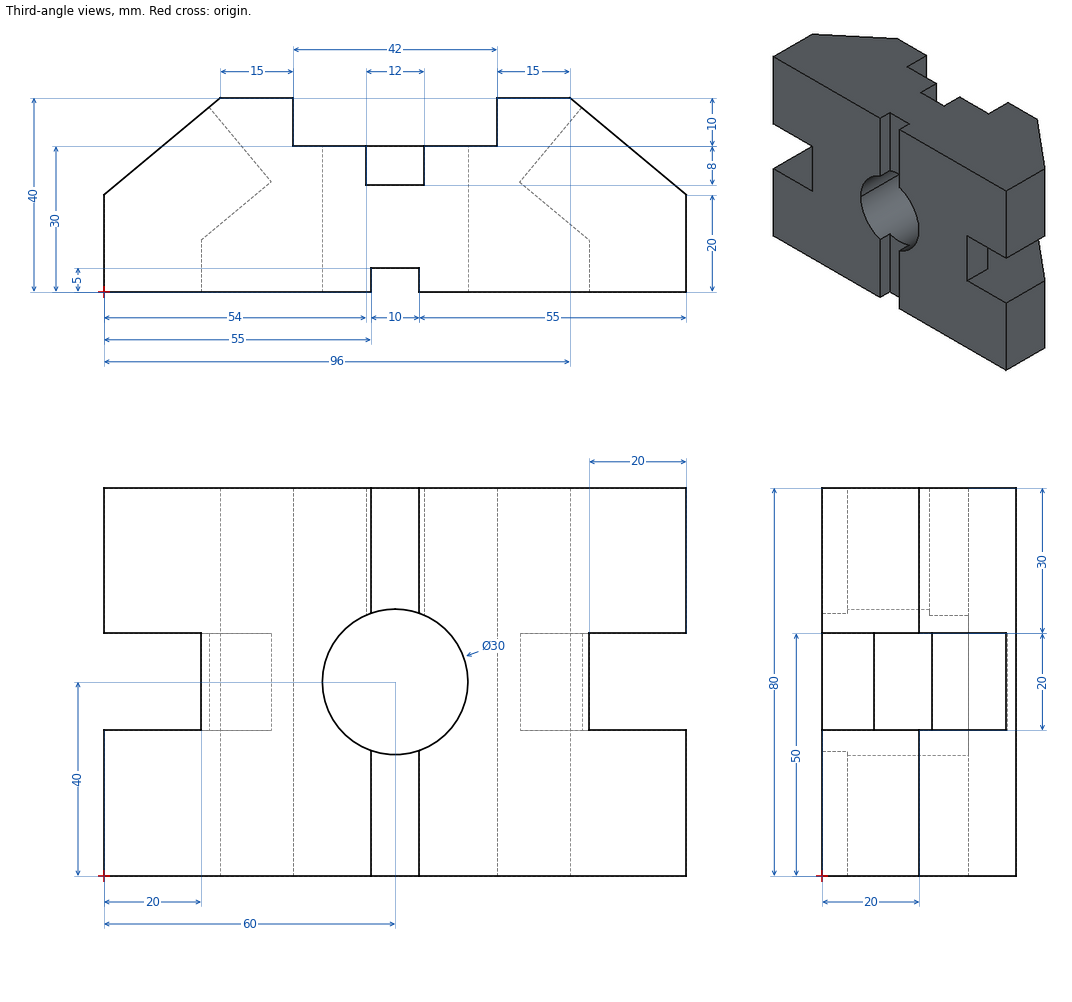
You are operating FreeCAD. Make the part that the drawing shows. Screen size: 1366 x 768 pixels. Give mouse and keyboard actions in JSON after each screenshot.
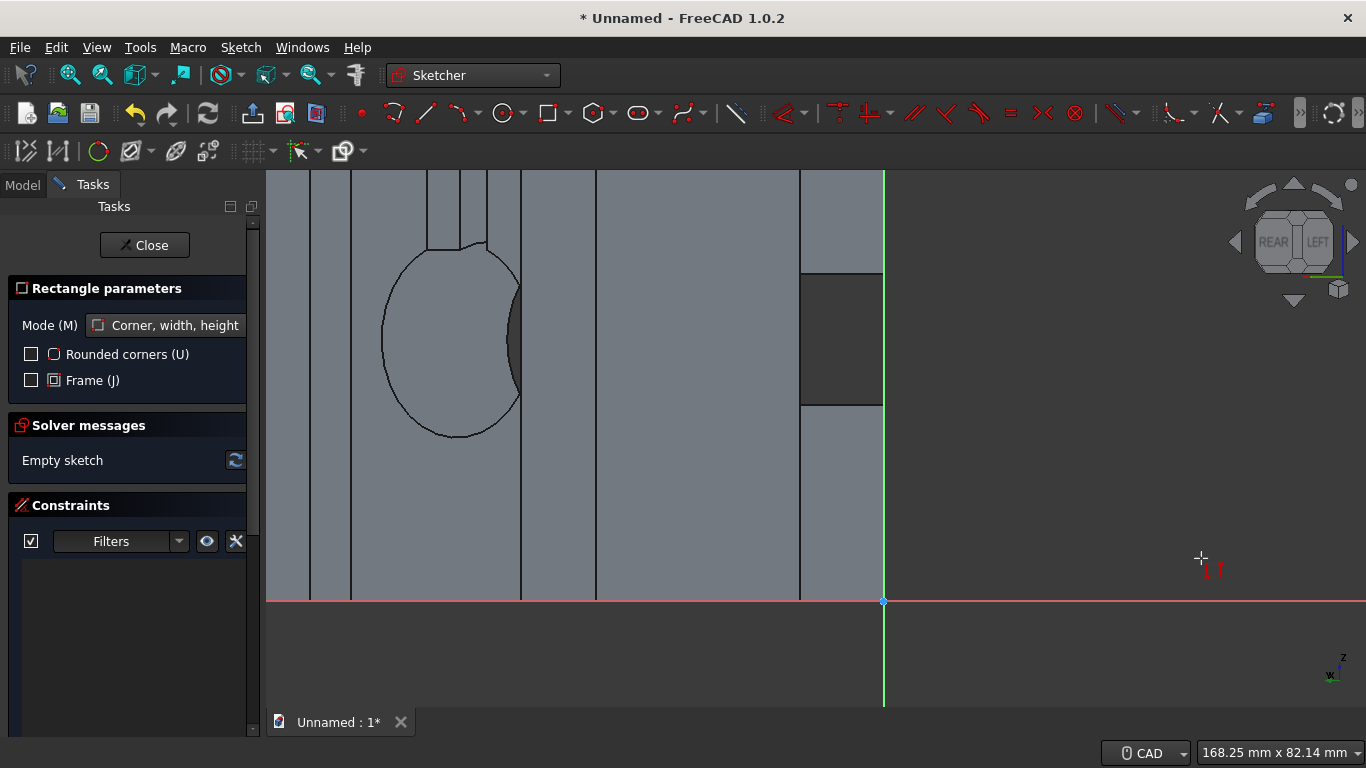
{"action": "left_click", "coordinate": [616, 274]}
{"action": "mouse_move", "coordinate": [800, 405]}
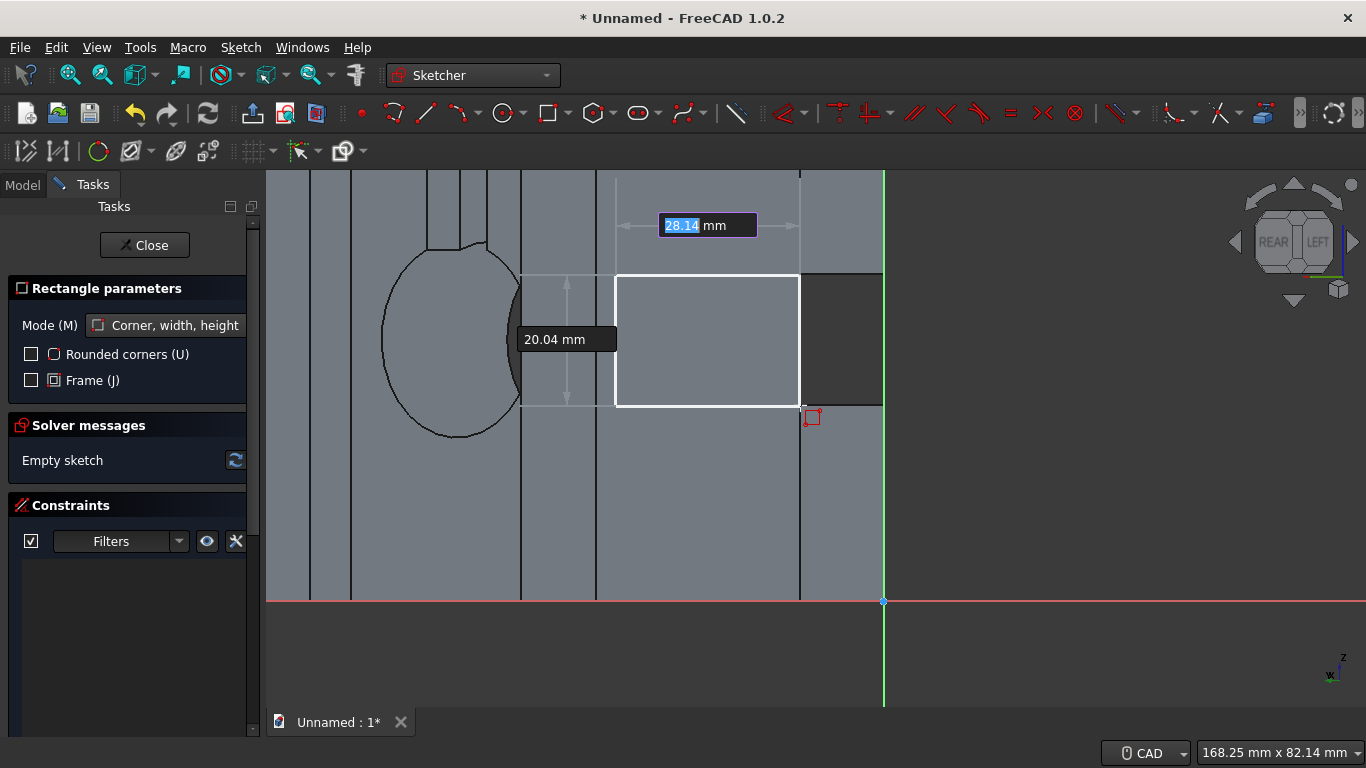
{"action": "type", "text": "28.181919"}
{"action": "key", "text": "Tab"}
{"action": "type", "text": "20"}
{"action": "key", "text": "Return"}
{"action": "key", "text": "Escape"}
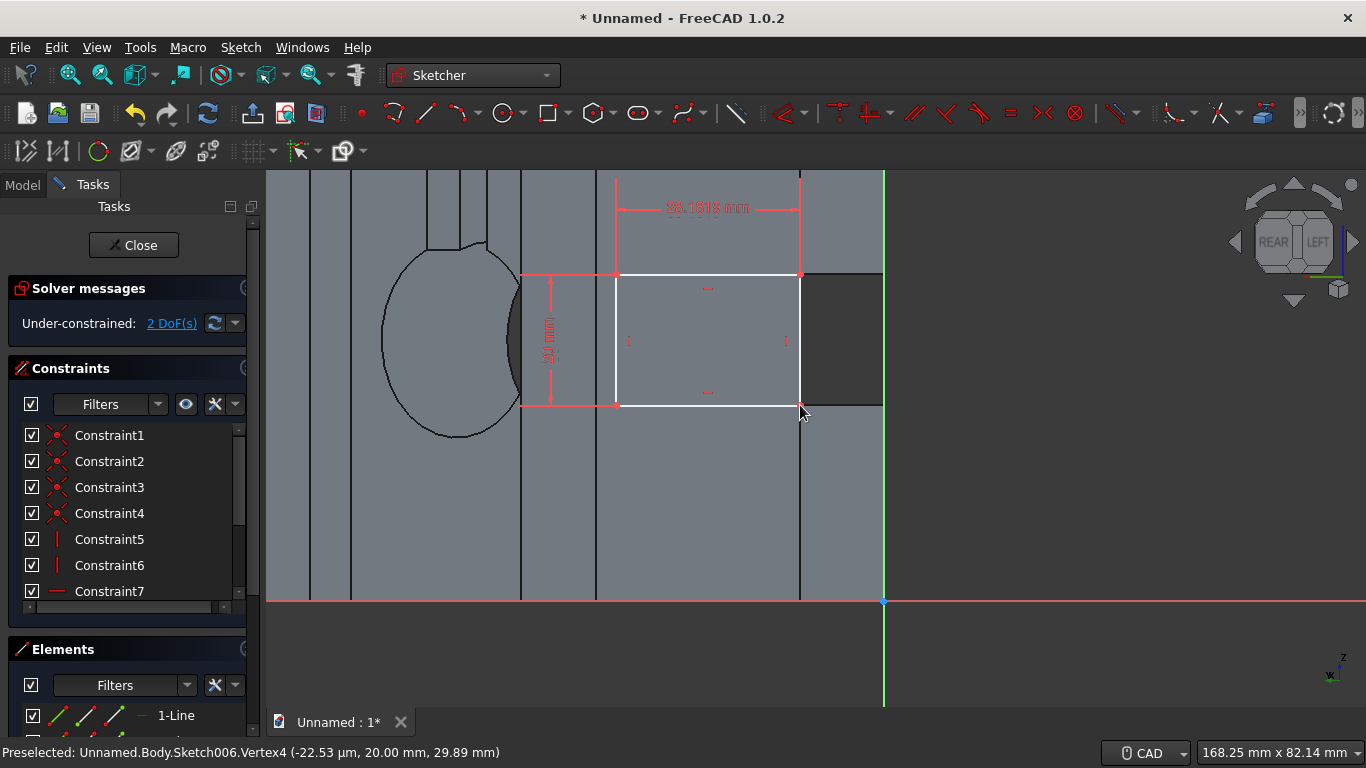
{"action": "left_click", "coordinate": [784, 114]}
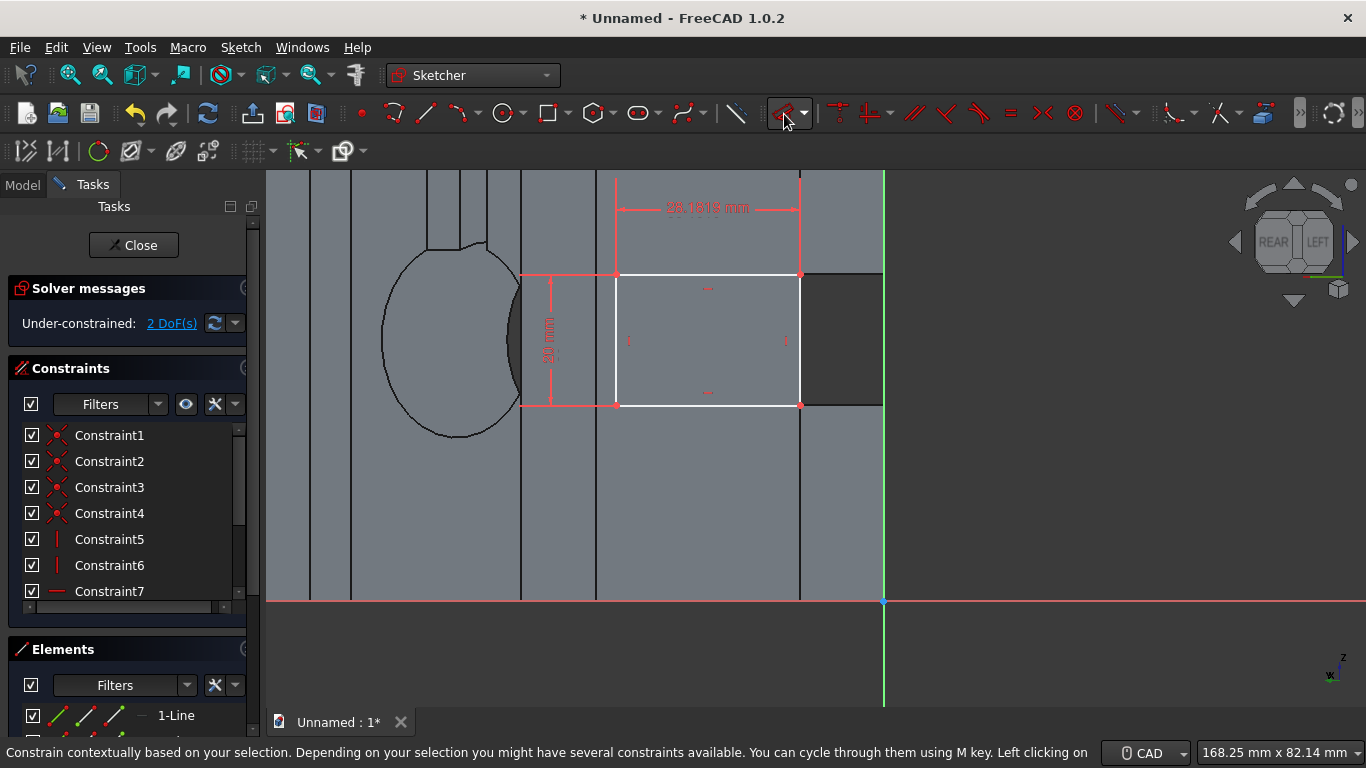
{"action": "left_click", "coordinate": [616, 275]}
{"action": "left_click", "coordinate": [918, 438]}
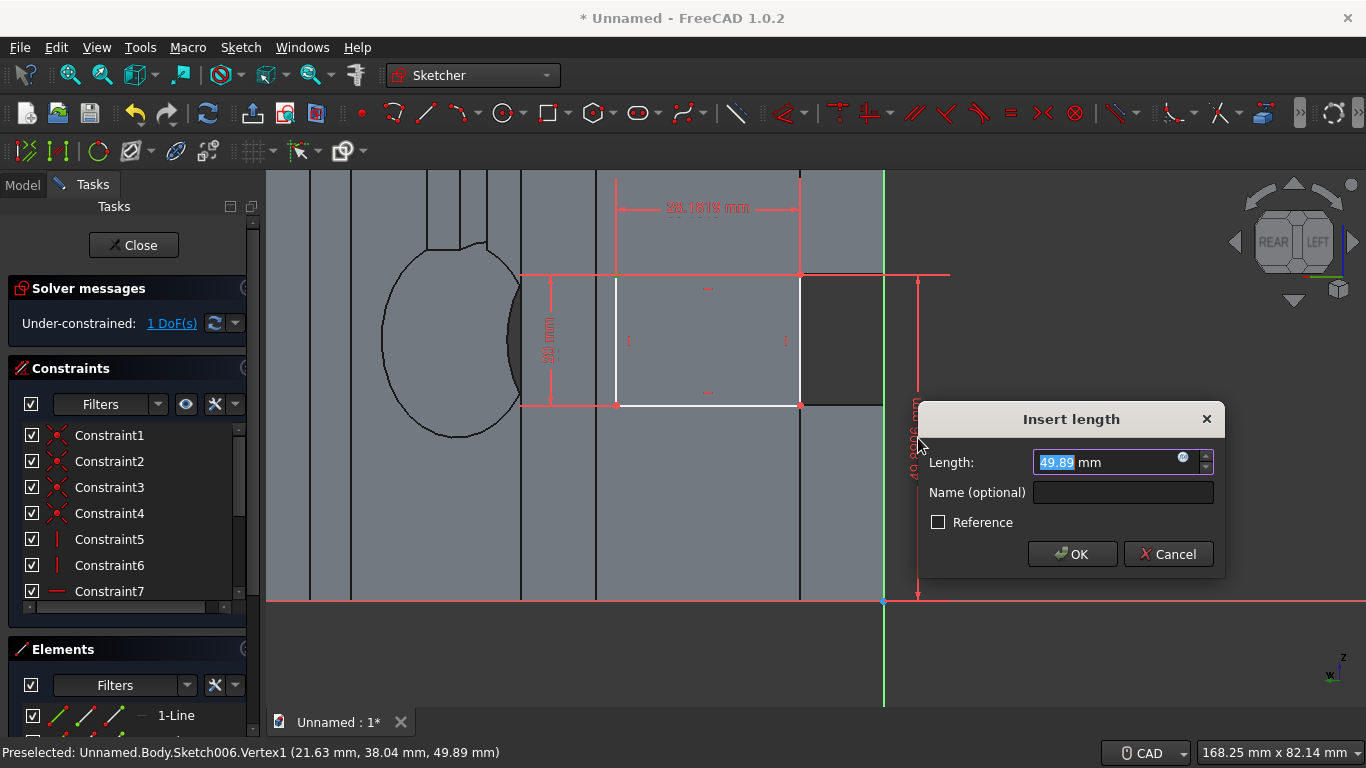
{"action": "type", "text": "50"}
{"action": "key", "text": "Return"}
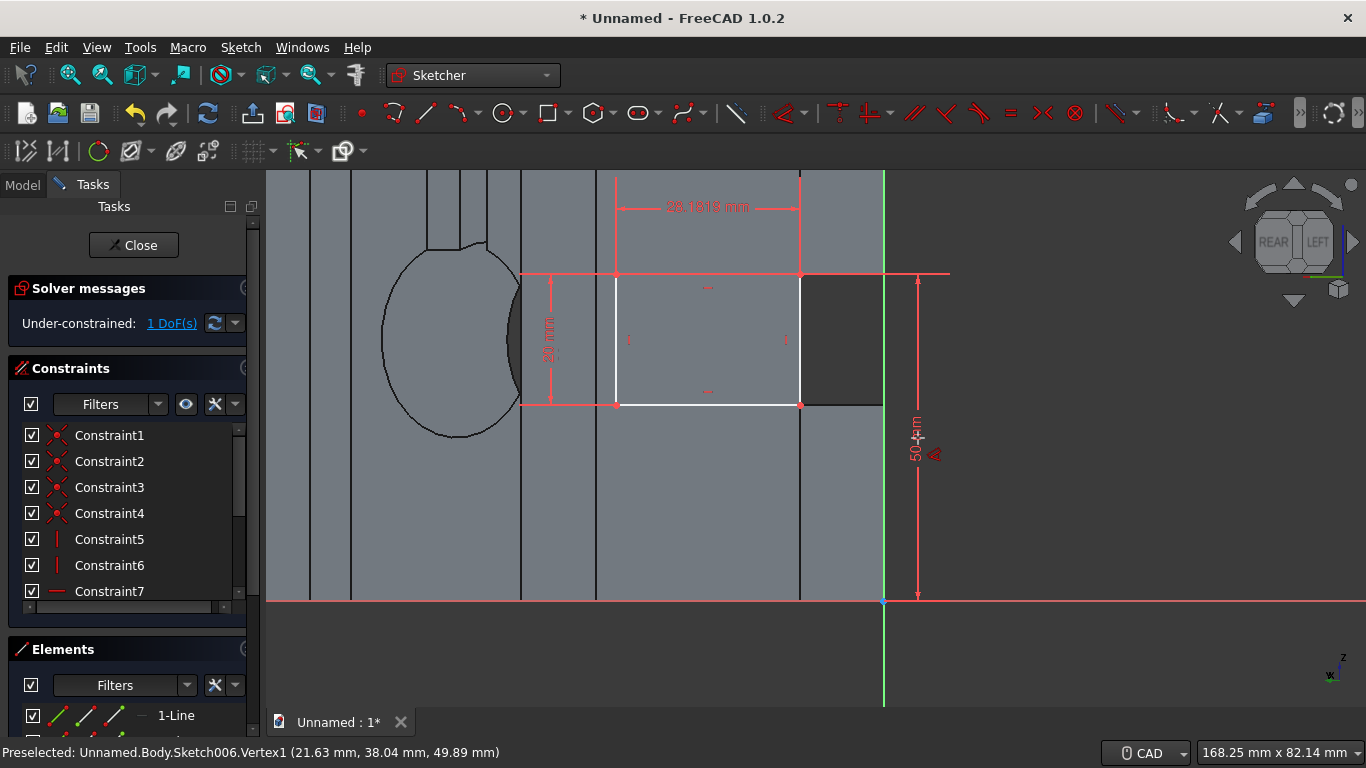
{"action": "left_click", "coordinate": [616, 274]}
{"action": "left_click", "coordinate": [750, 635]}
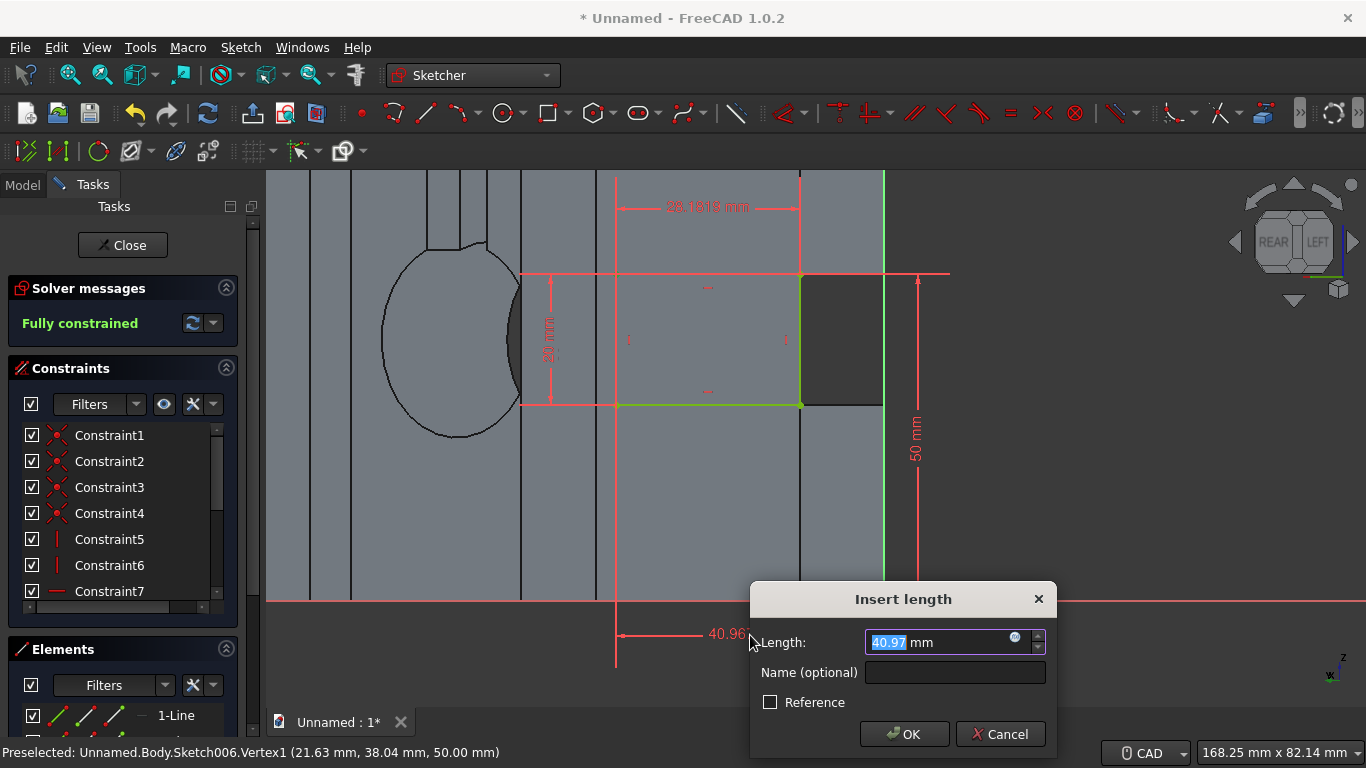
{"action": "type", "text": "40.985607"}
{"action": "key", "text": "Return"}
{"action": "key", "text": "Escape"}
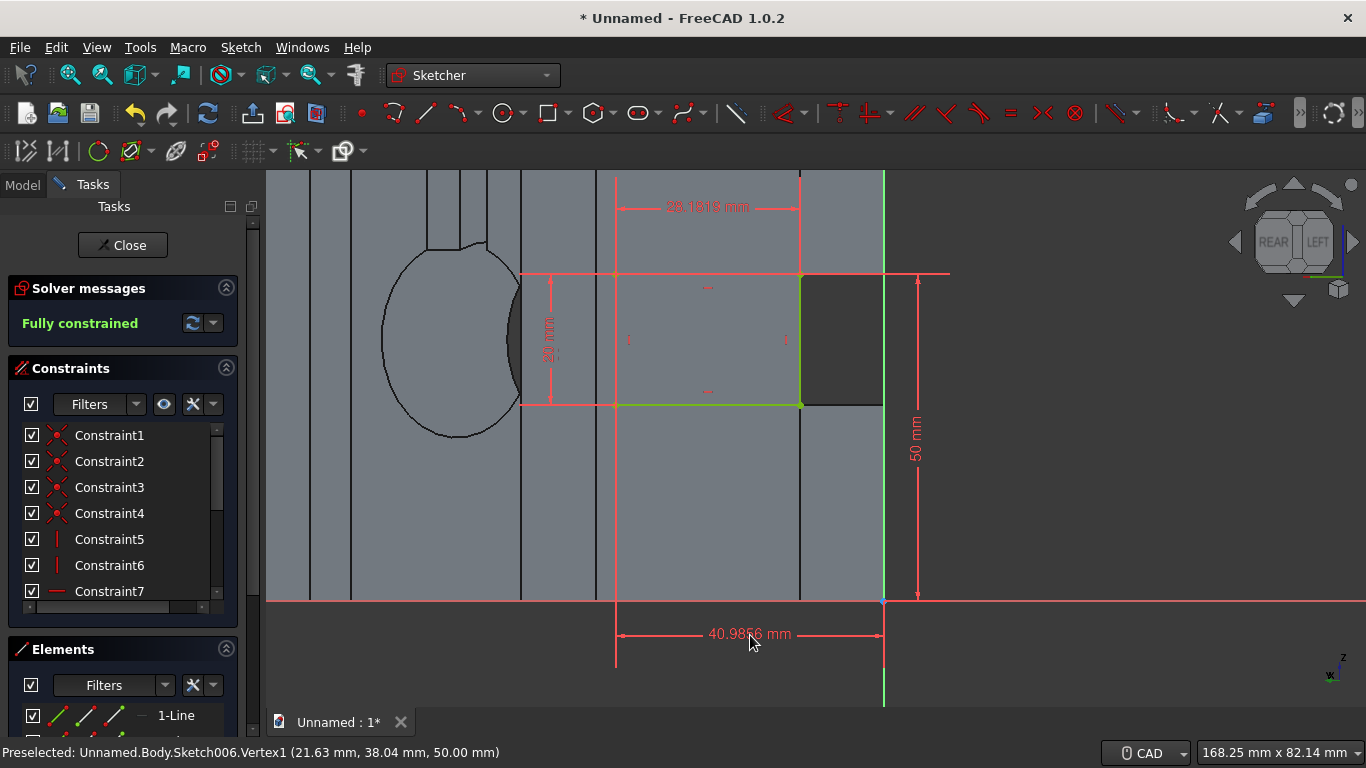
{"action": "left_click", "coordinate": [123, 245]}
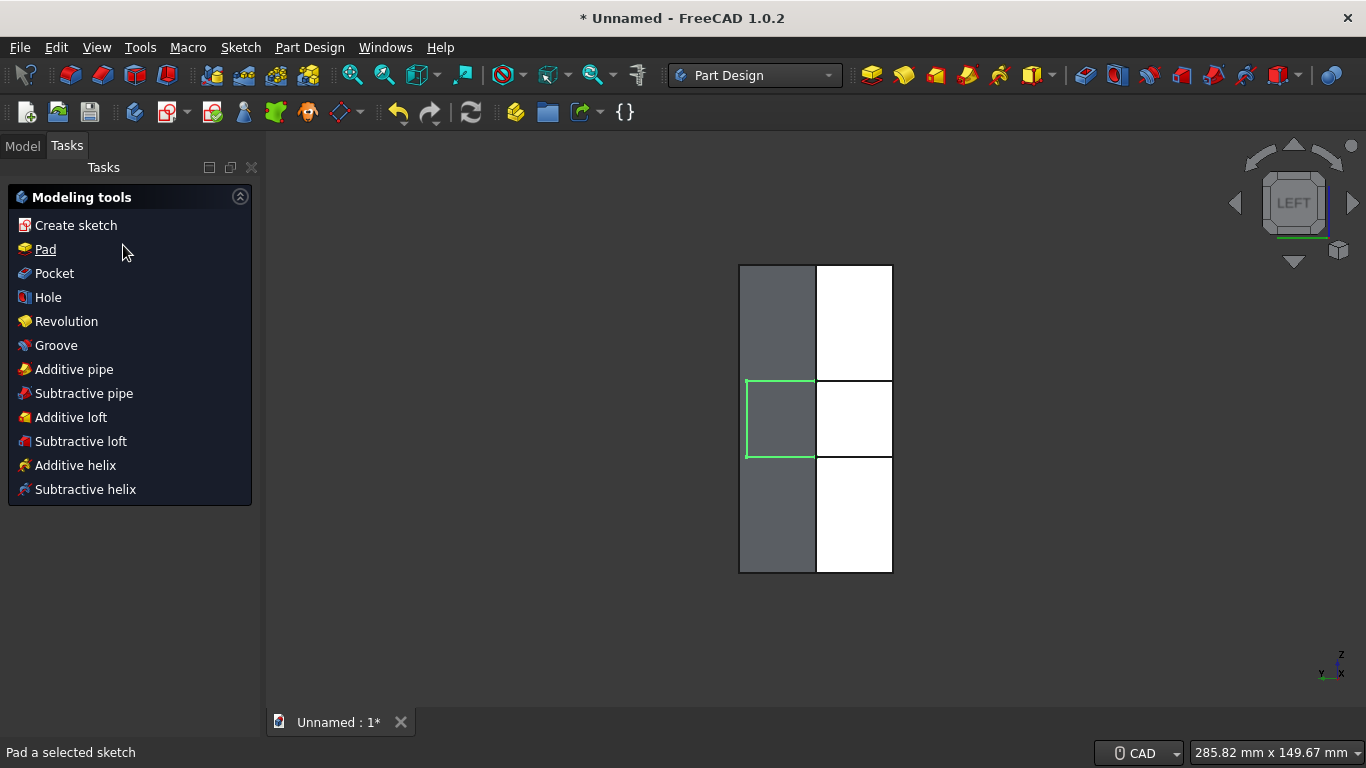
{"action": "left_click", "coordinate": [1086, 76]}